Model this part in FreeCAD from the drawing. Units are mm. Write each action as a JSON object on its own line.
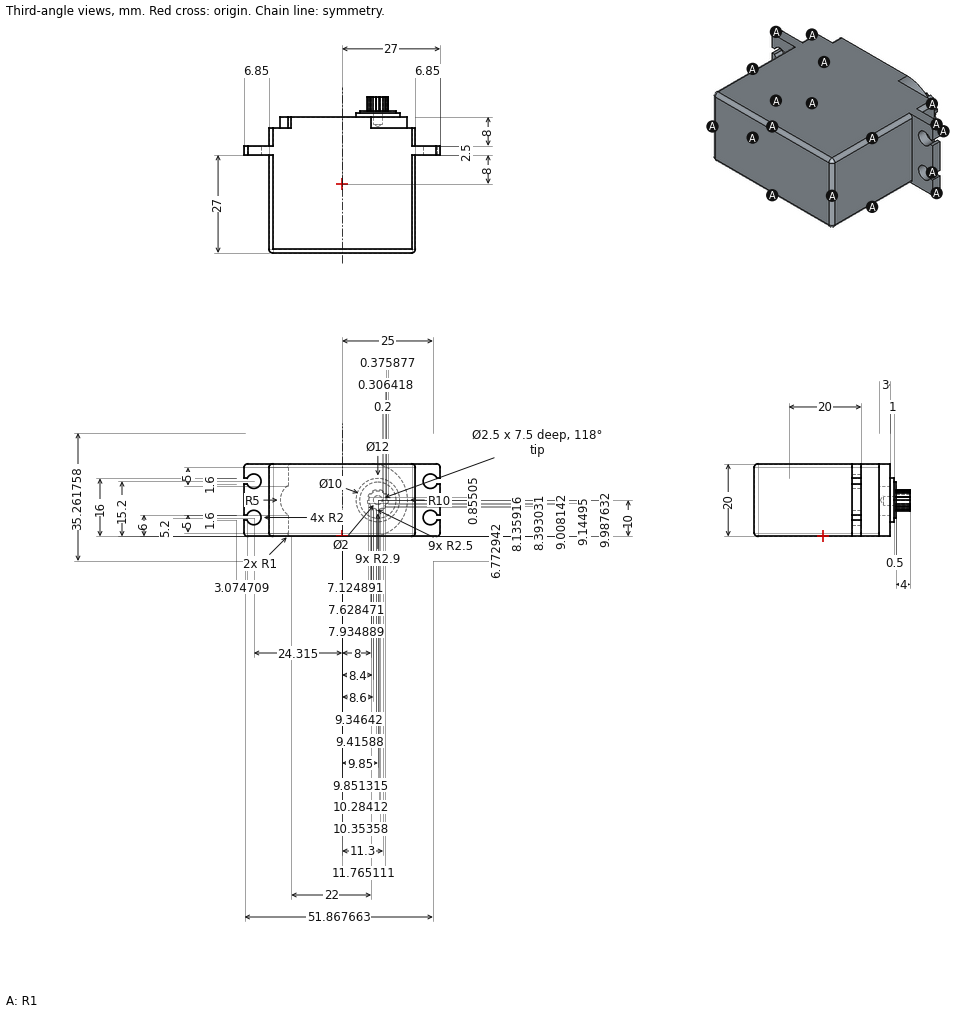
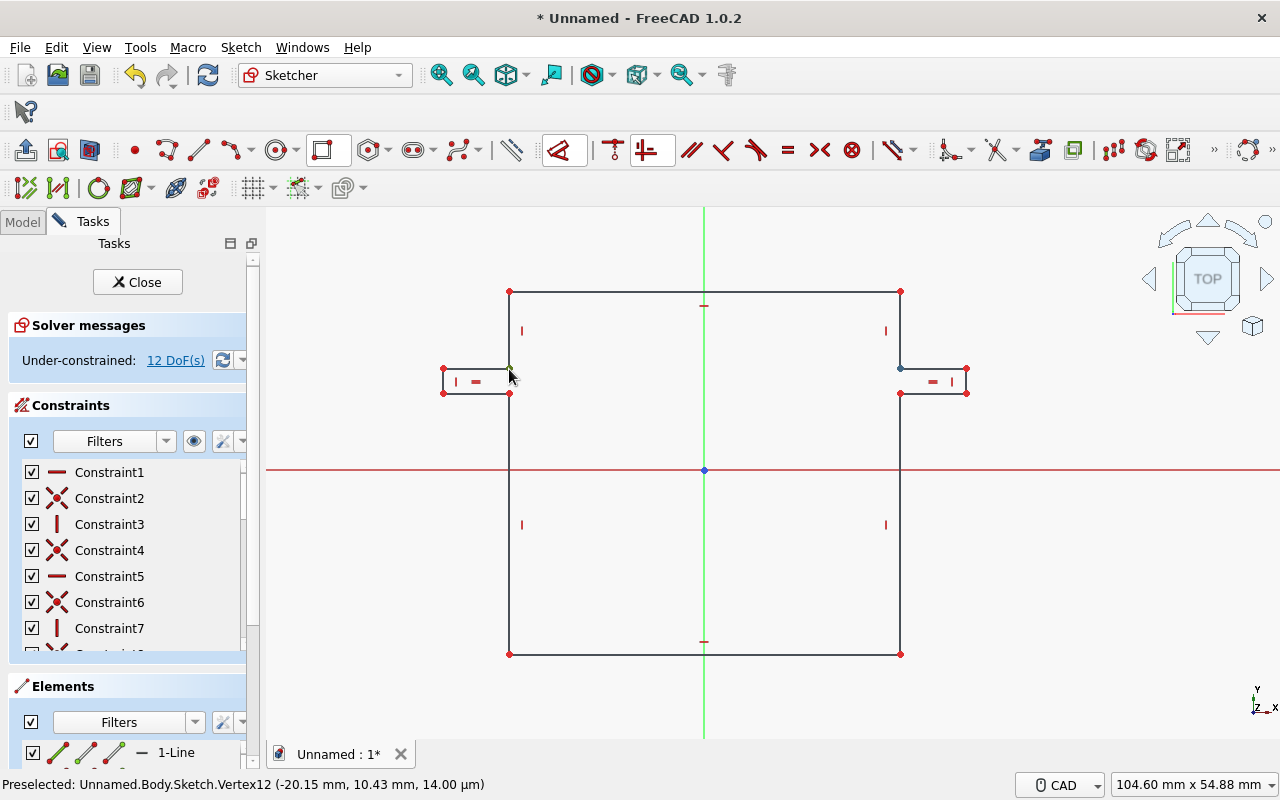
{"action": "left_click", "coordinate": [704, 609]}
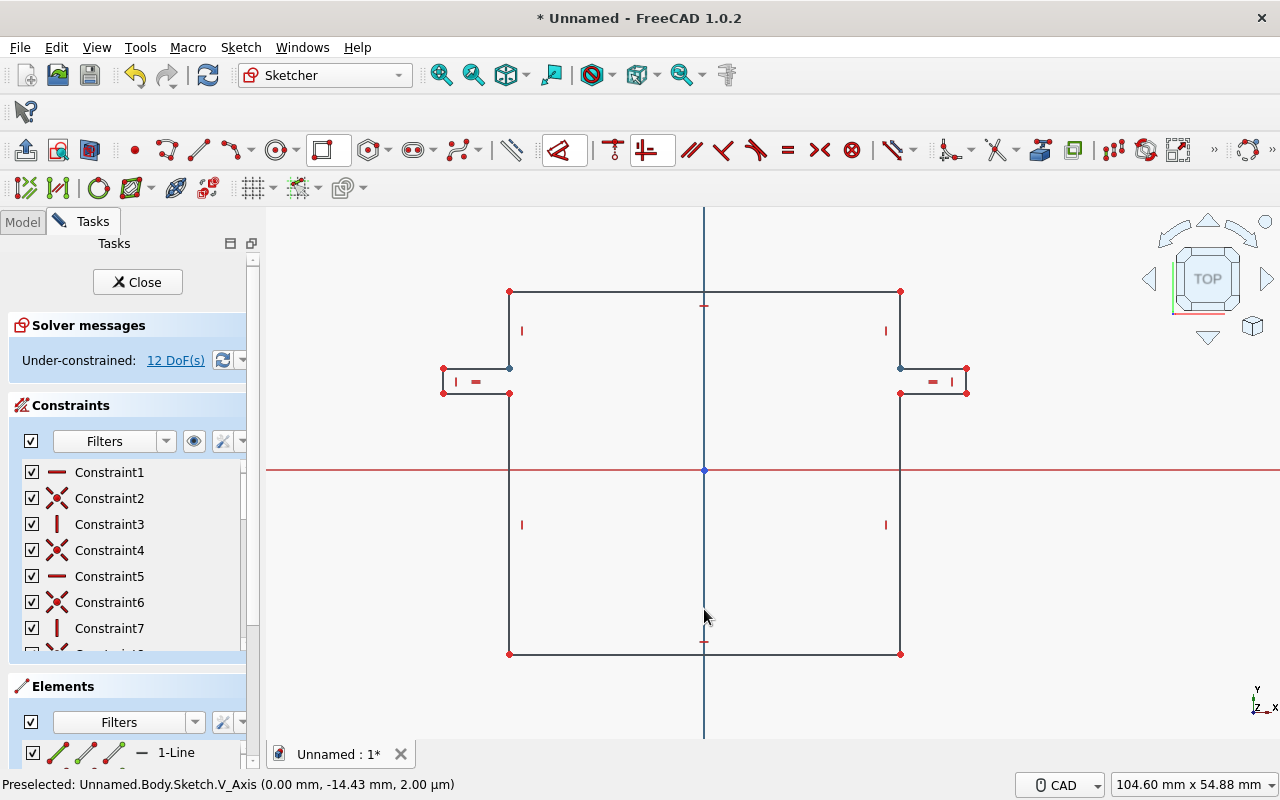
{"action": "left_click", "coordinate": [820, 150]}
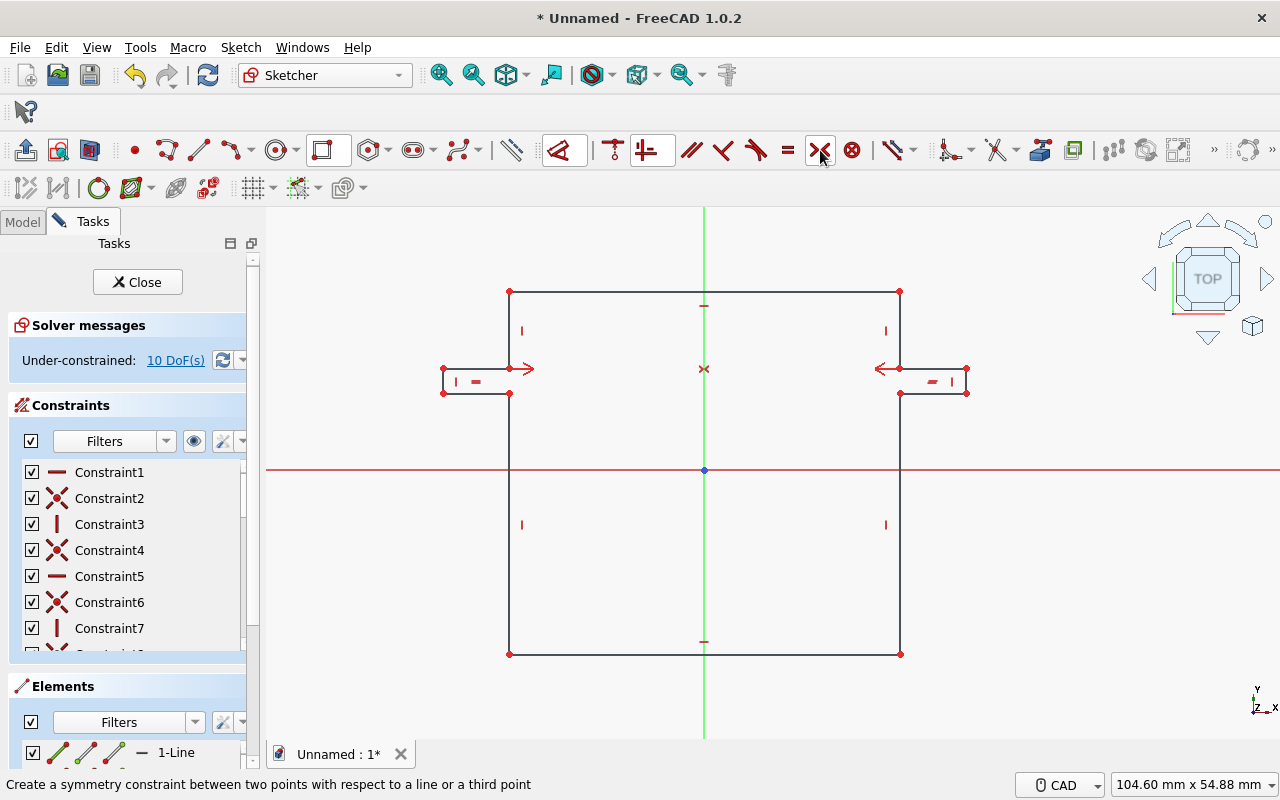
{"action": "left_click", "coordinate": [966, 394]}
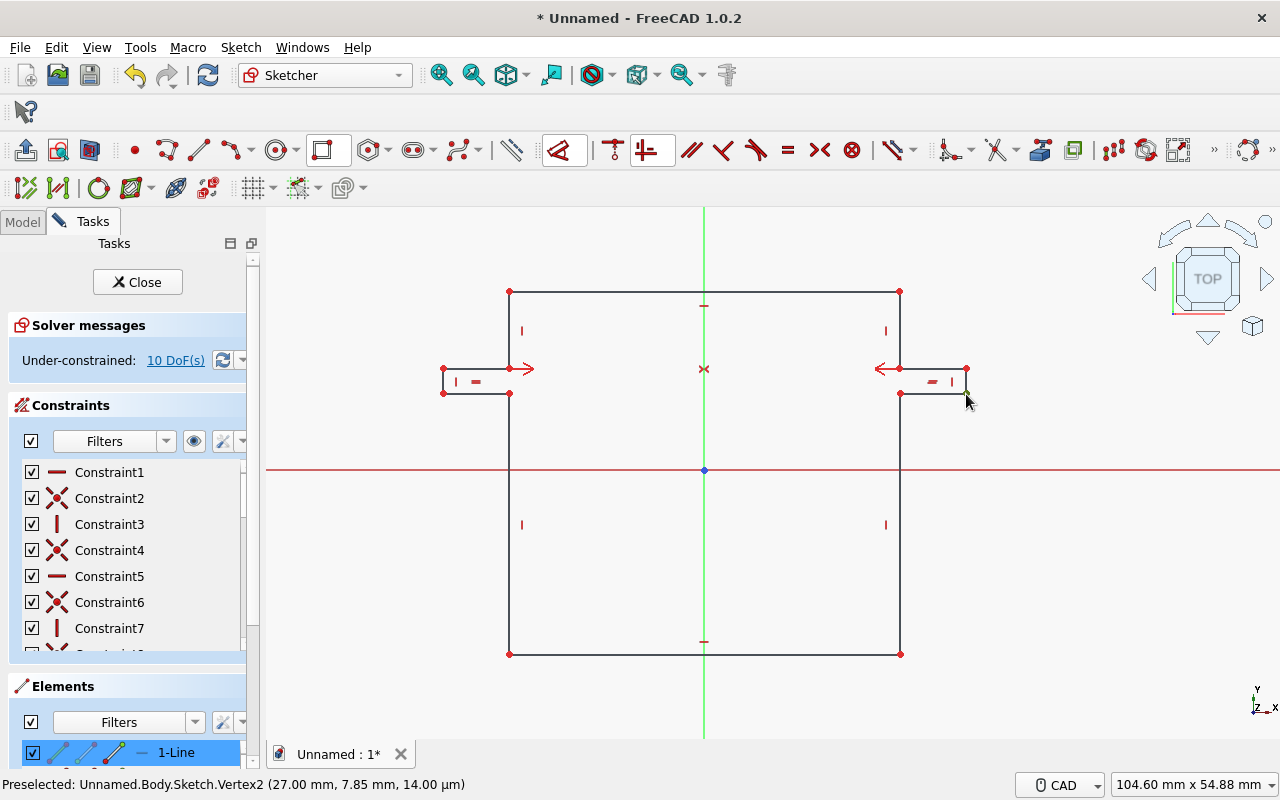
{"action": "left_click", "coordinate": [443, 394]}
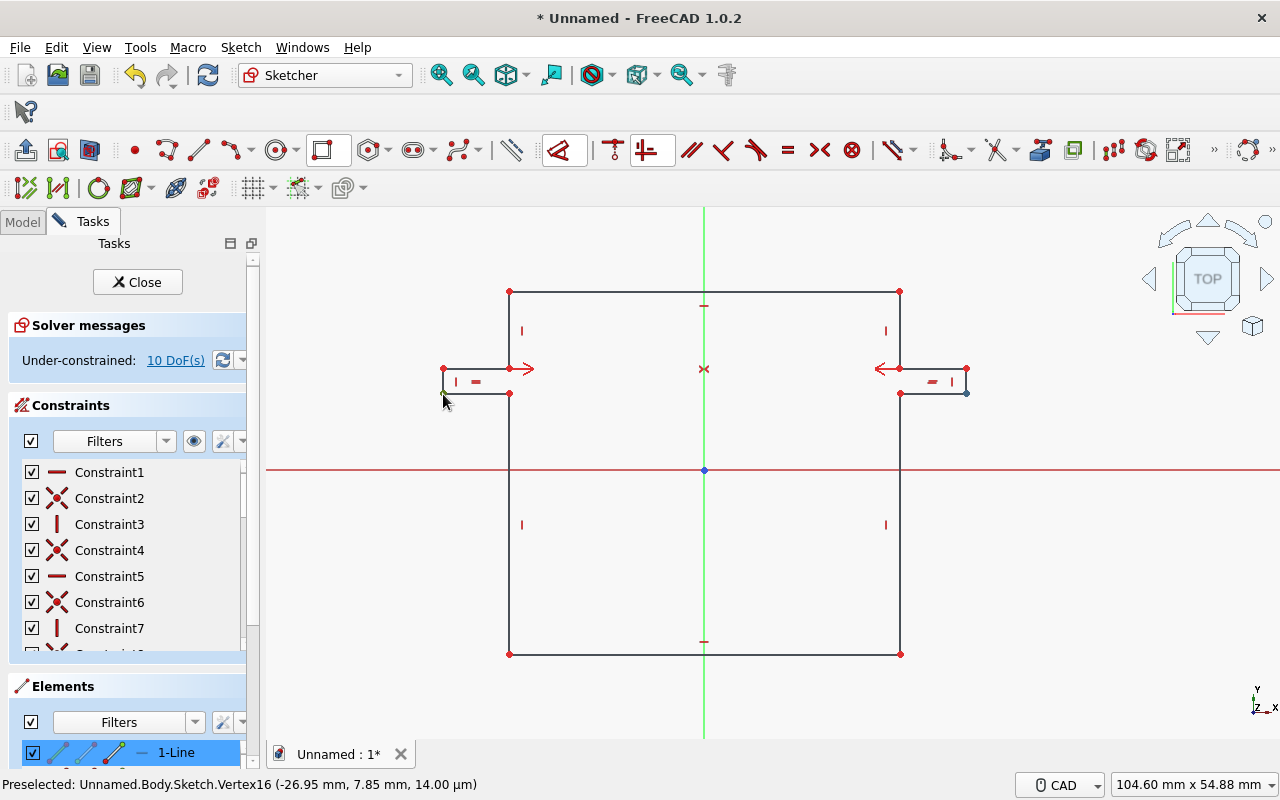
{"action": "left_click", "coordinate": [704, 609]}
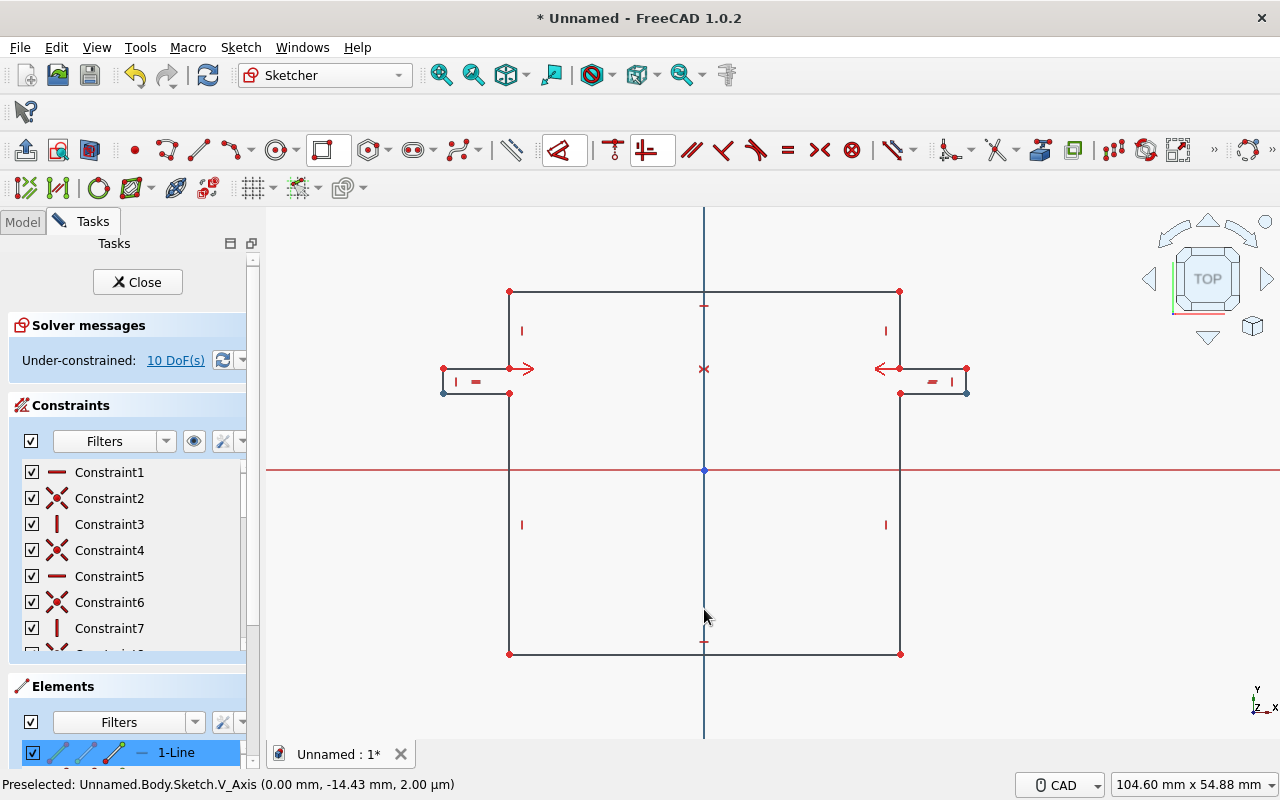
{"action": "left_click", "coordinate": [820, 150]}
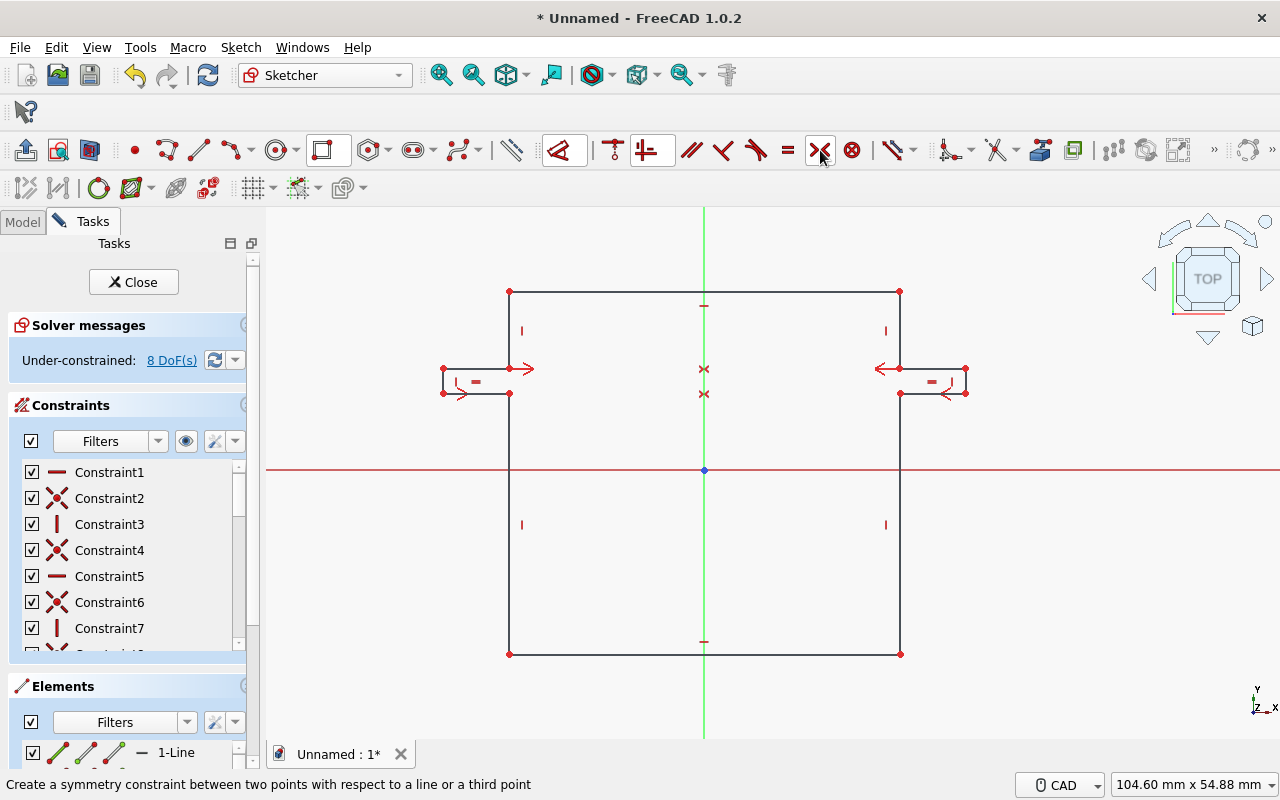
{"action": "left_click", "coordinate": [558, 150]}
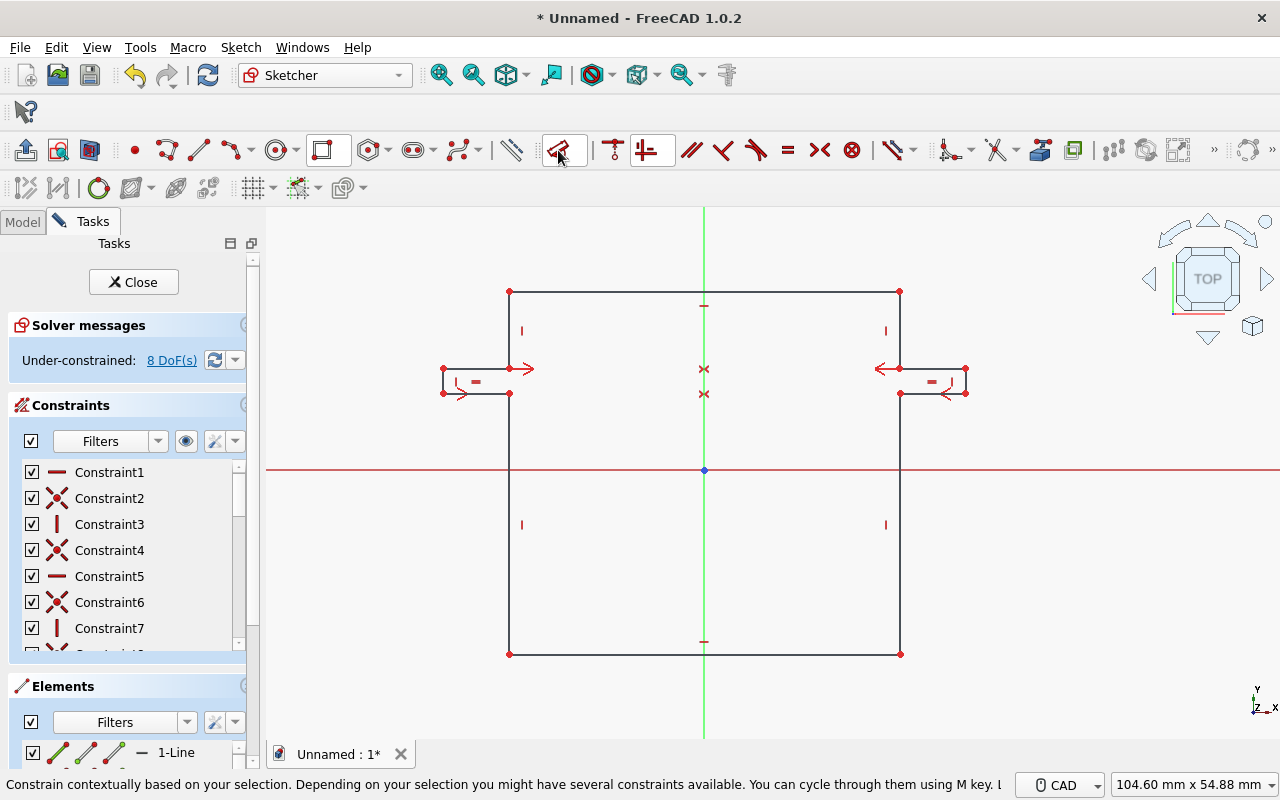
{"action": "left_click", "coordinate": [900, 346]}
{"action": "left_click", "coordinate": [934, 330]}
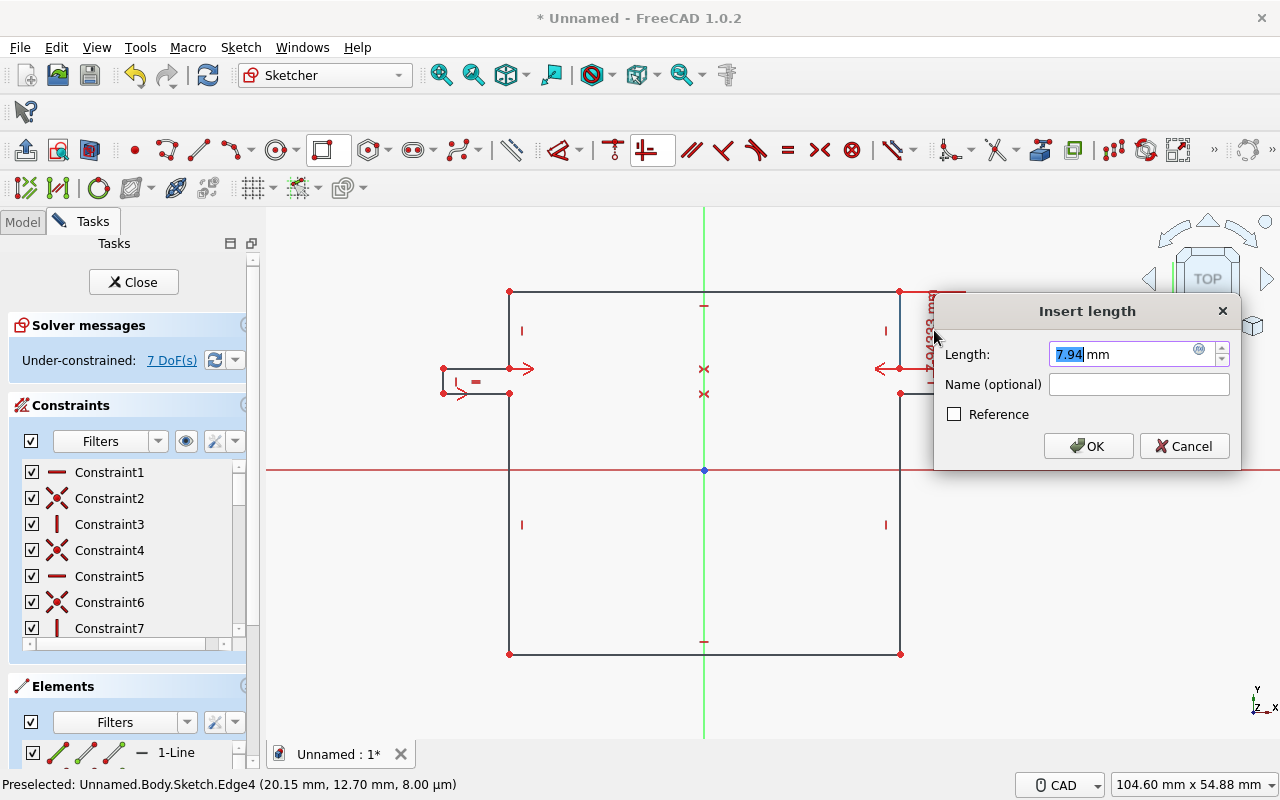
{"action": "type", "text": "8"}
{"action": "key", "text": "Return"}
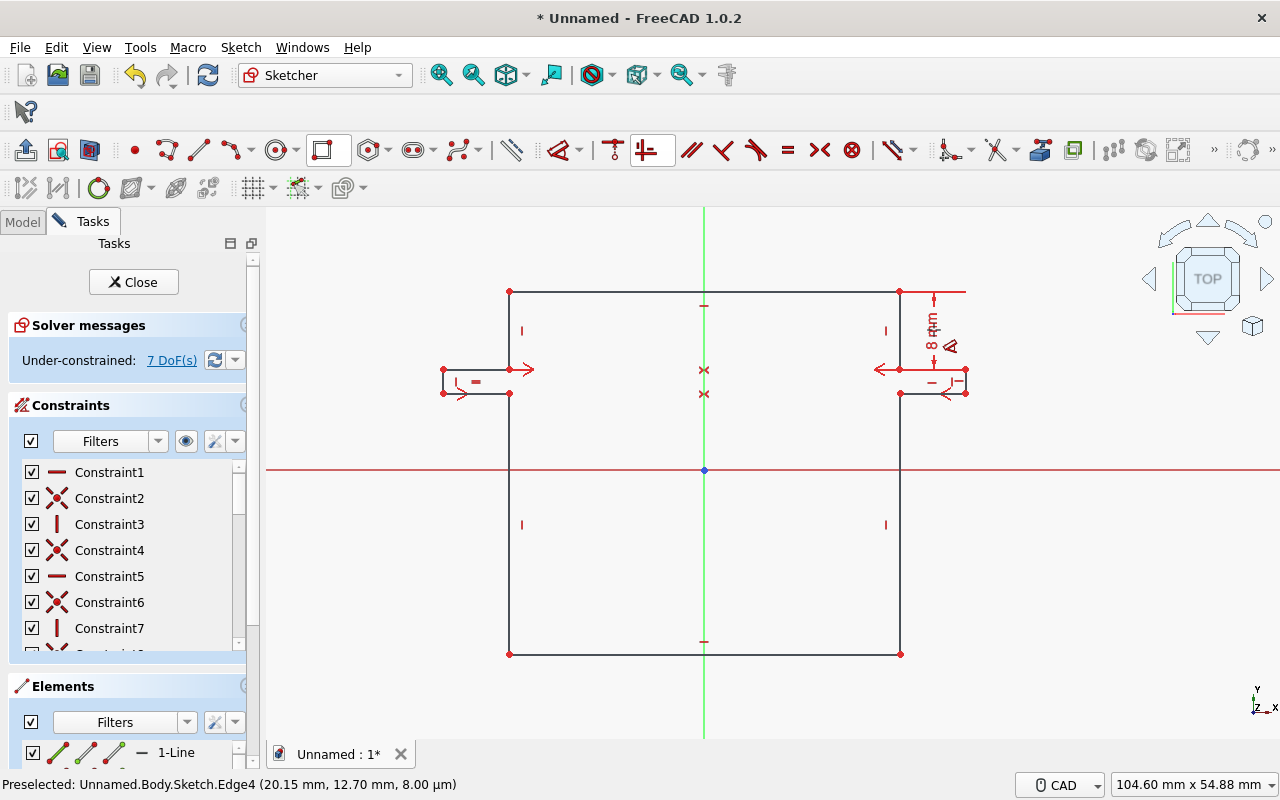
{"action": "left_click", "coordinate": [509, 472]}
{"action": "left_click", "coordinate": [475, 524]}